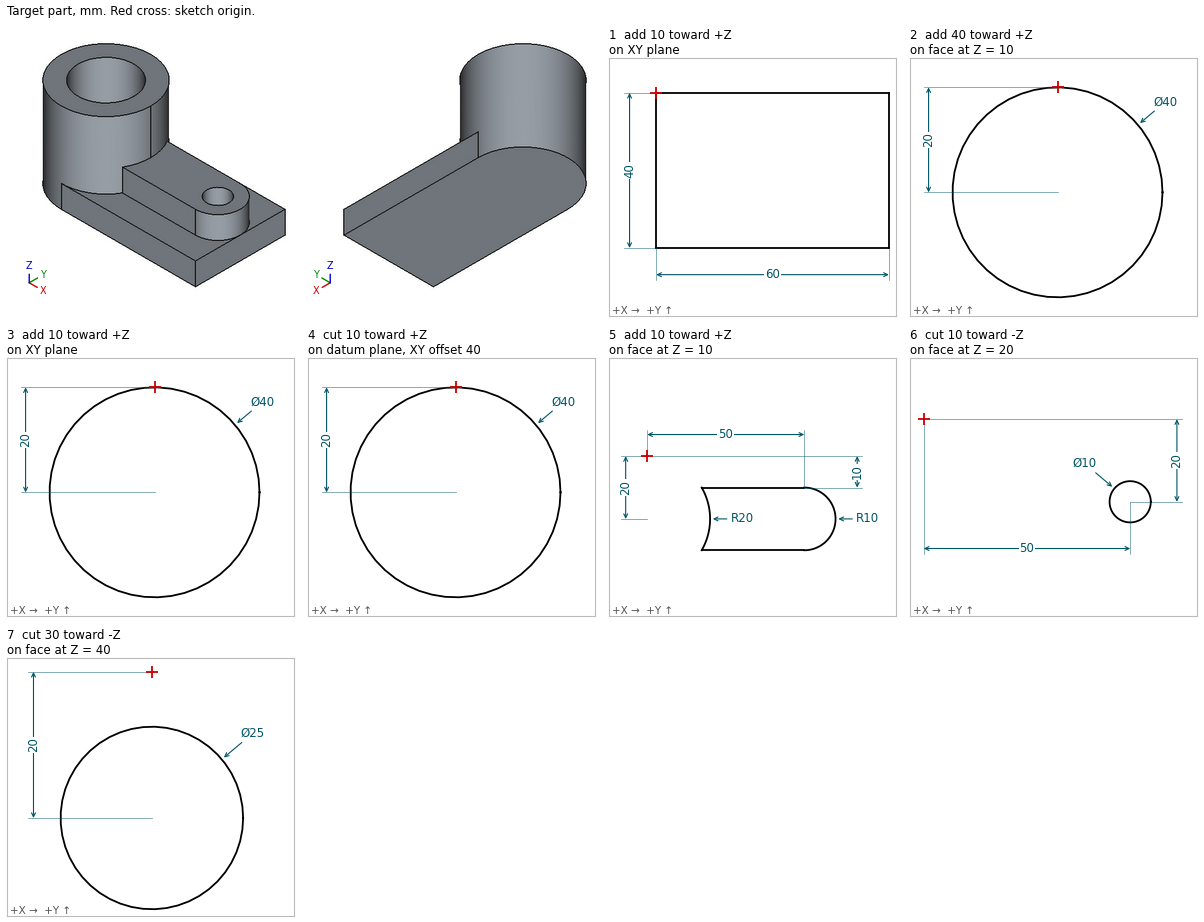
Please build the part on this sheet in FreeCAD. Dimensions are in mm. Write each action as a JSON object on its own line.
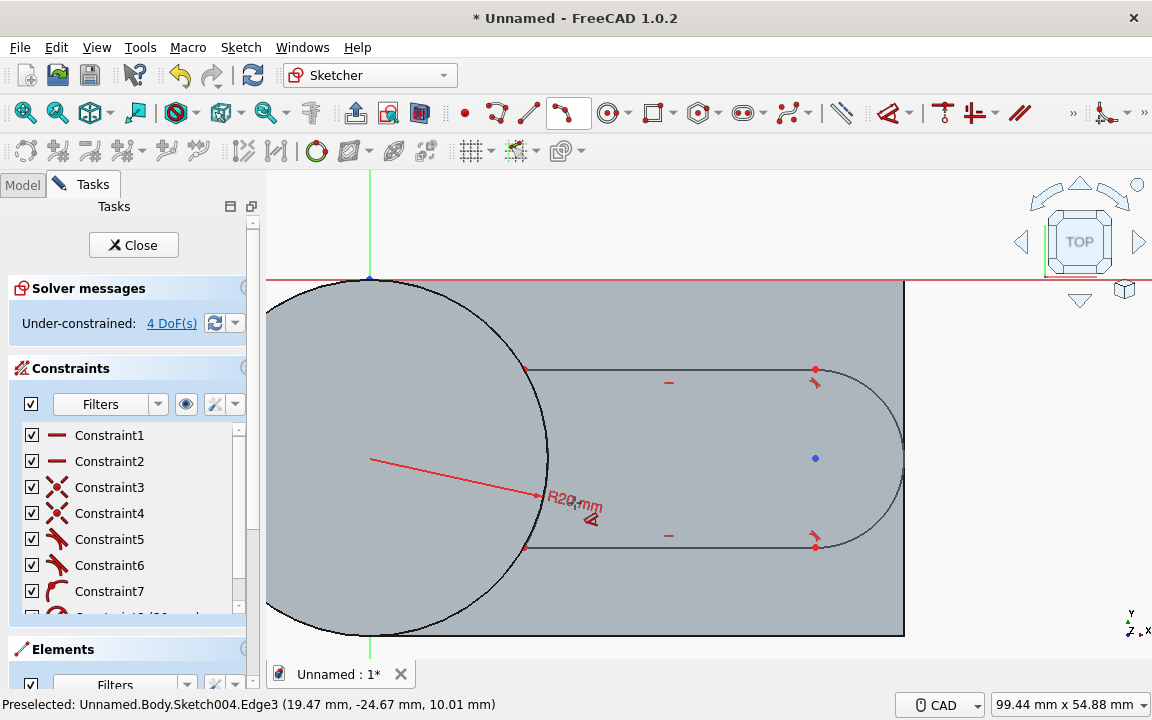
{"action": "left_click", "coordinate": [887, 511]}
{"action": "left_click", "coordinate": [913, 530]}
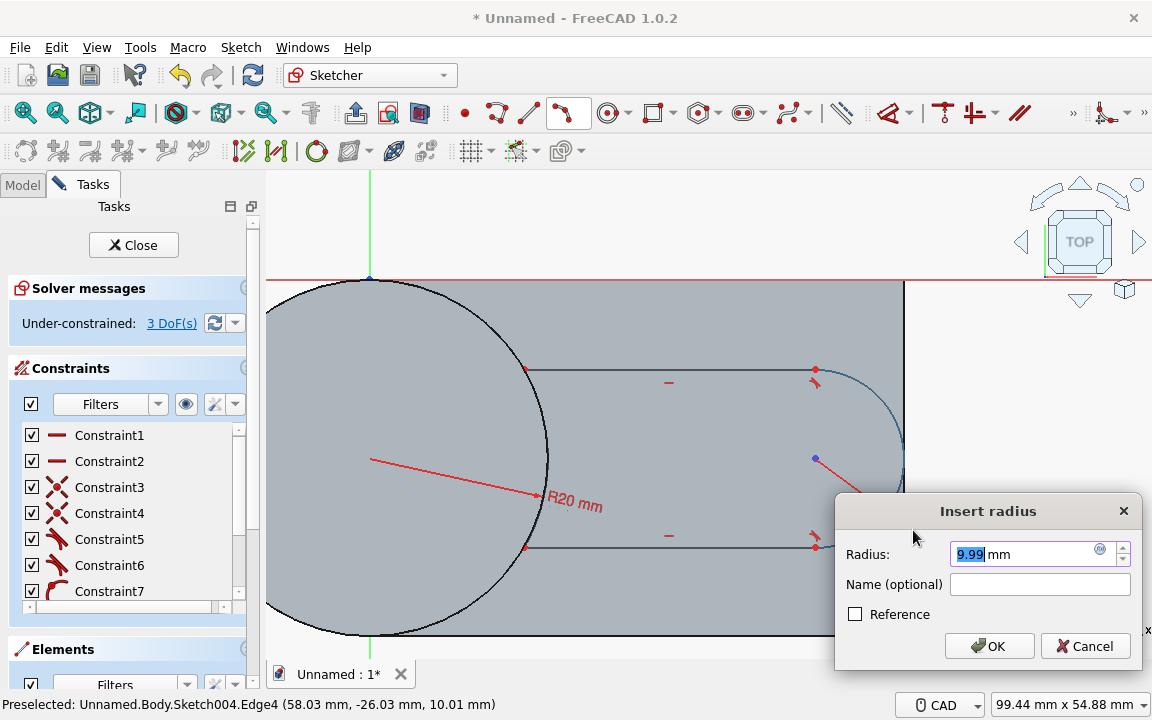
{"action": "type", "text": "10"}
{"action": "key", "text": "Return"}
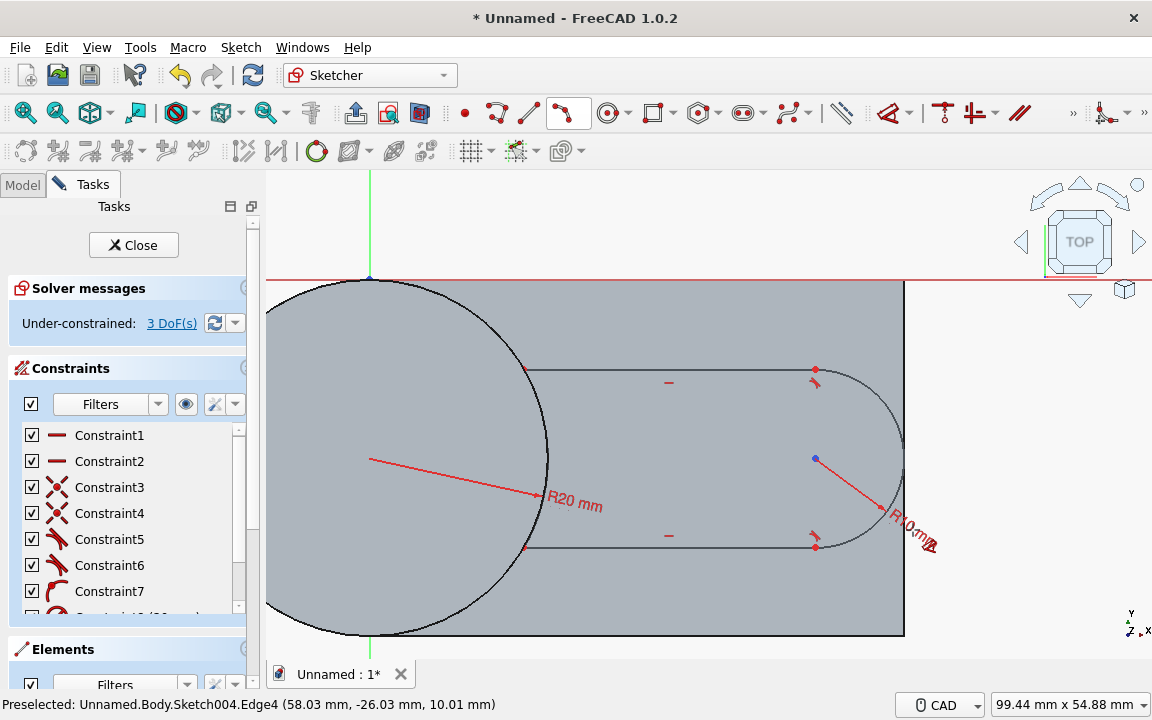
{"action": "left_click", "coordinate": [815, 370]}
{"action": "left_click", "coordinate": [592, 246]}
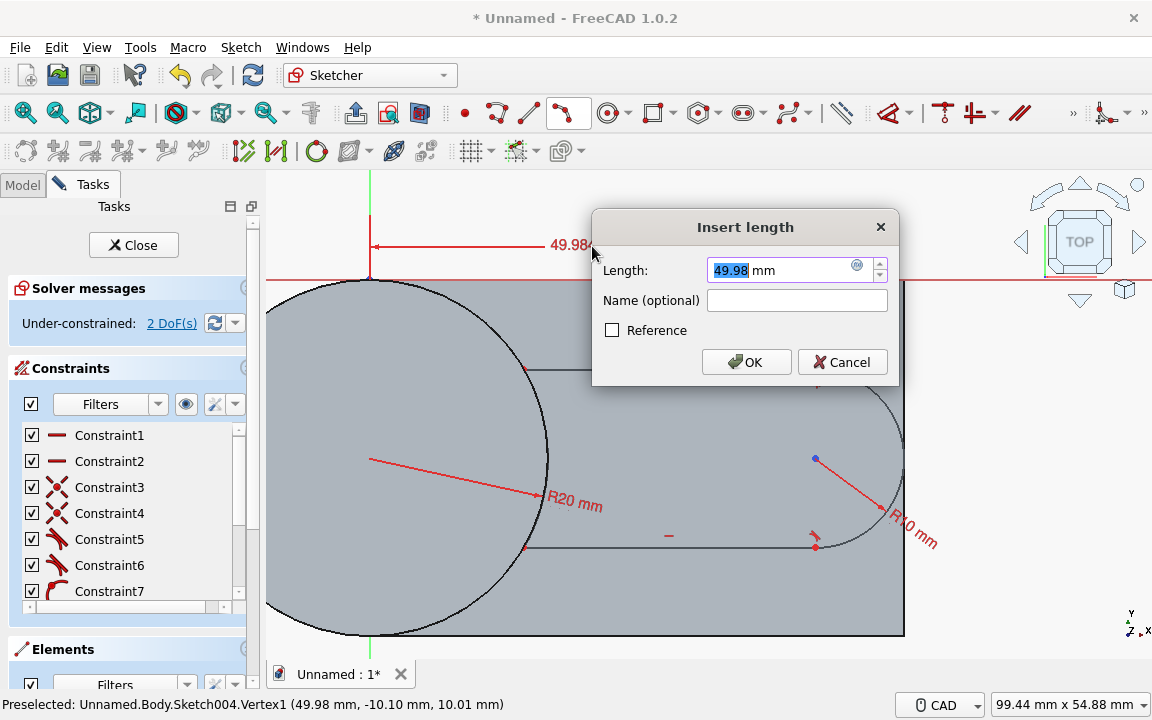
{"action": "type", "text": "50"}
{"action": "key", "text": "Return"}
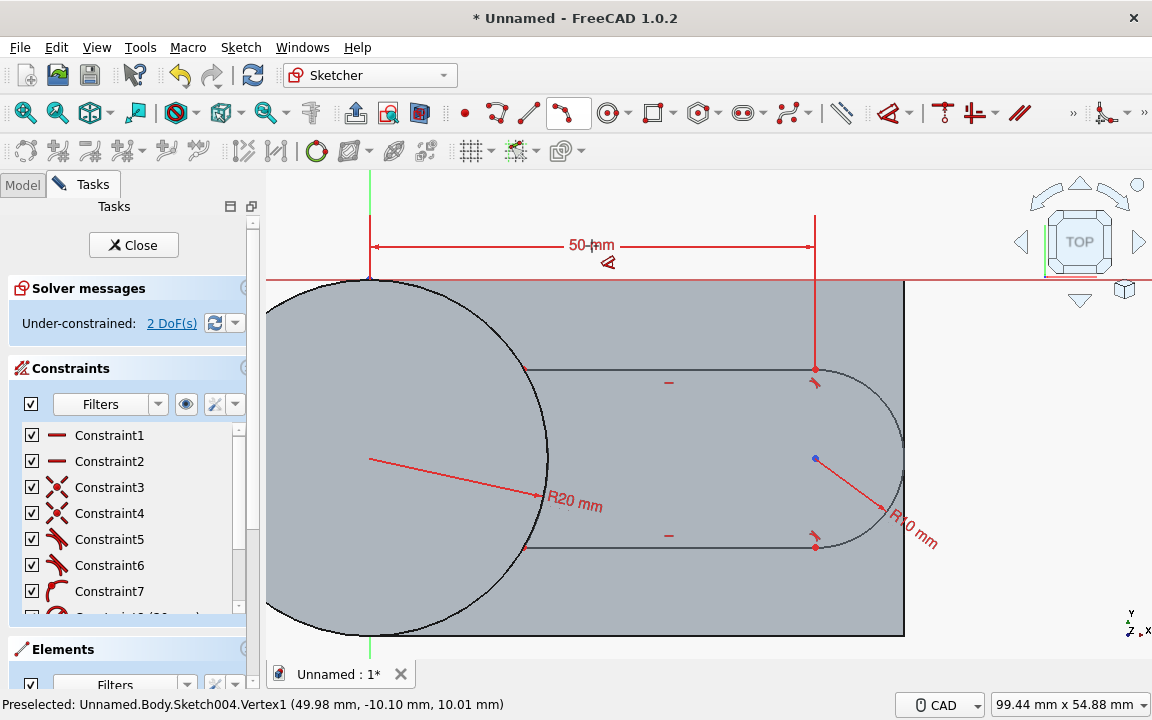
{"action": "left_click", "coordinate": [815, 370]}
{"action": "left_click", "coordinate": [336, 325]}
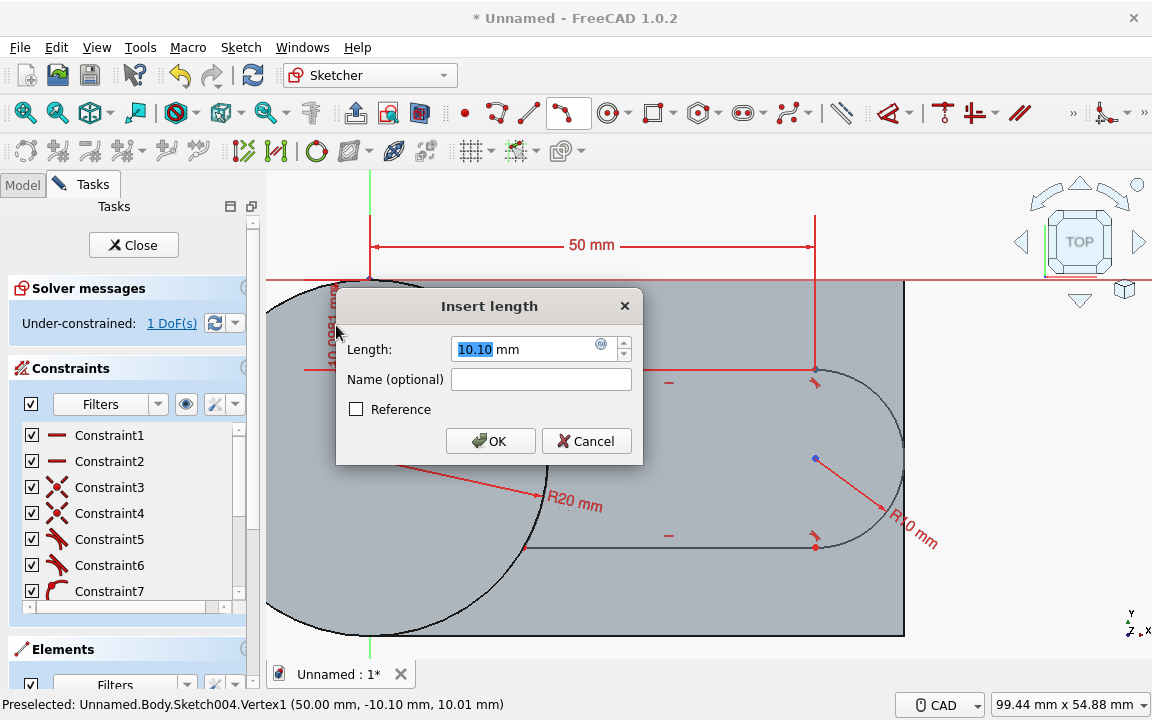
{"action": "type", "text": "10"}
{"action": "key", "text": "Return"}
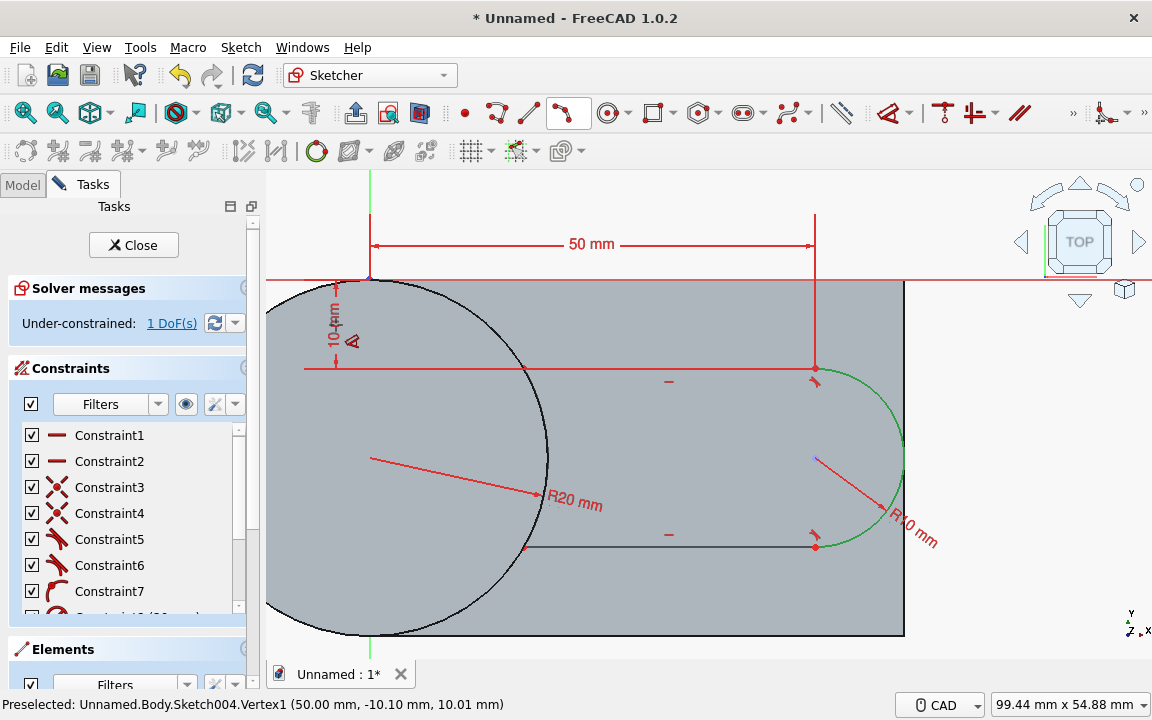
{"action": "left_click", "coordinate": [370, 458]}
{"action": "left_click", "coordinate": [336, 369]}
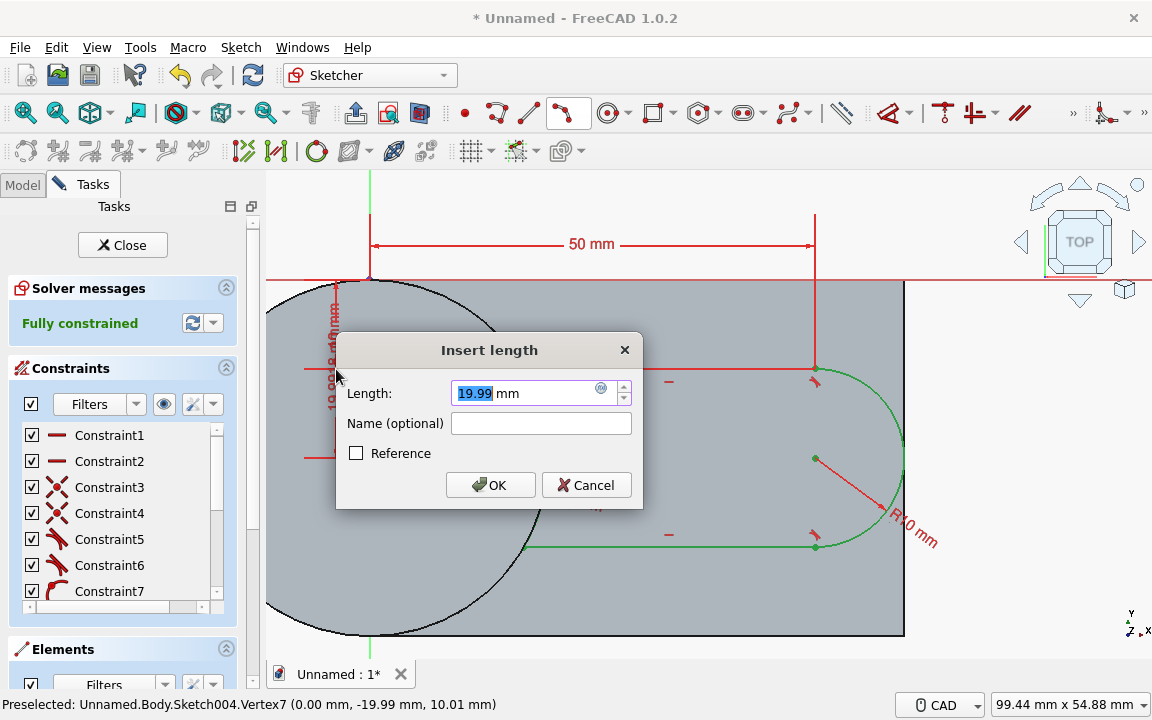
{"action": "type", "text": "20"}
{"action": "key", "text": "Return"}
{"action": "key", "text": "Escape"}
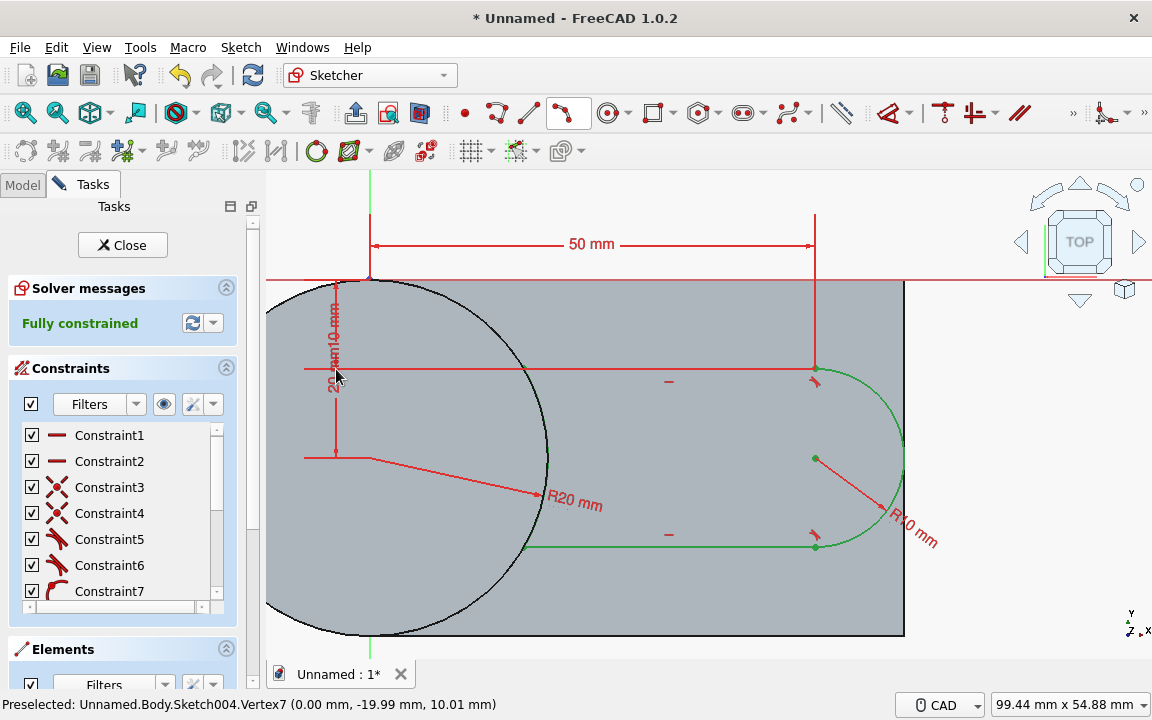
{"action": "left_click", "coordinate": [123, 245]}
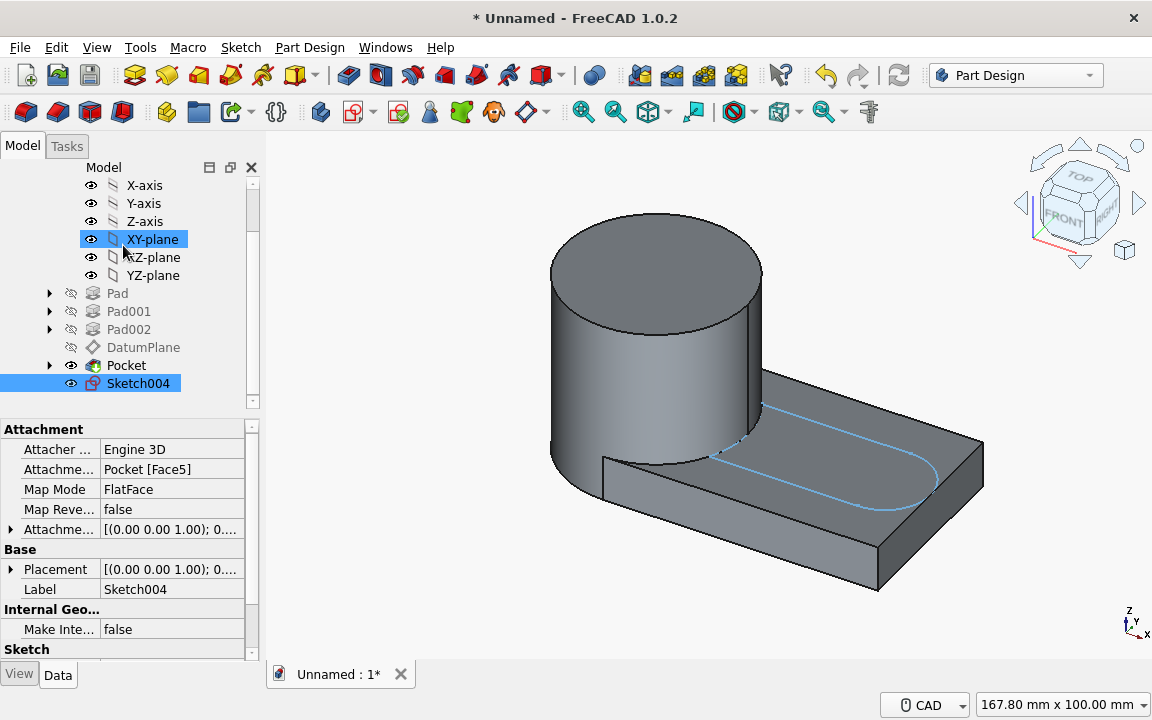
{"action": "left_click", "coordinate": [136, 76]}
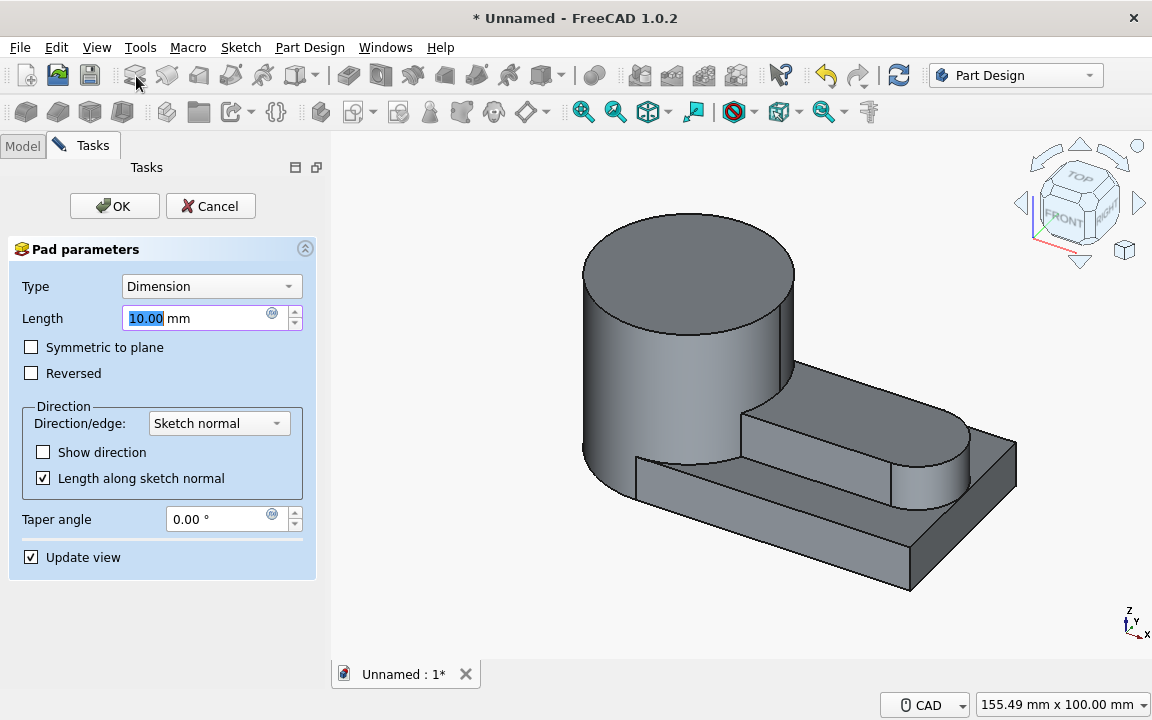
{"action": "type", "text": "10"}
{"action": "key", "text": "Tab"}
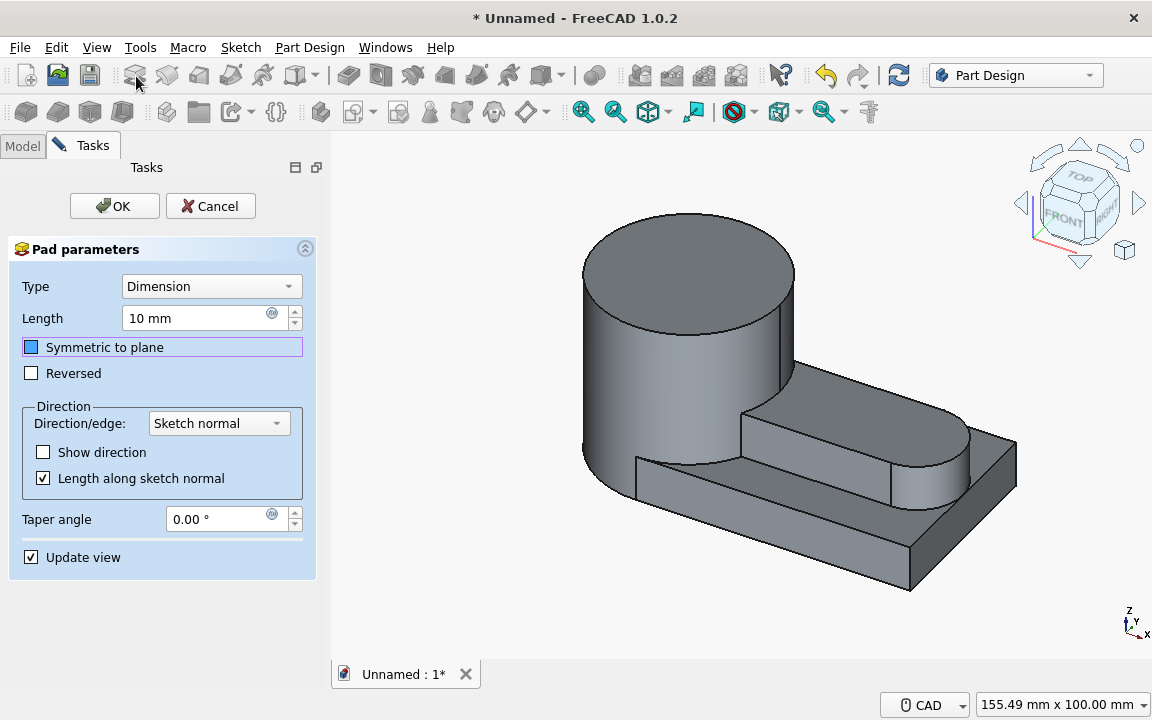
{"action": "left_click", "coordinate": [115, 206]}